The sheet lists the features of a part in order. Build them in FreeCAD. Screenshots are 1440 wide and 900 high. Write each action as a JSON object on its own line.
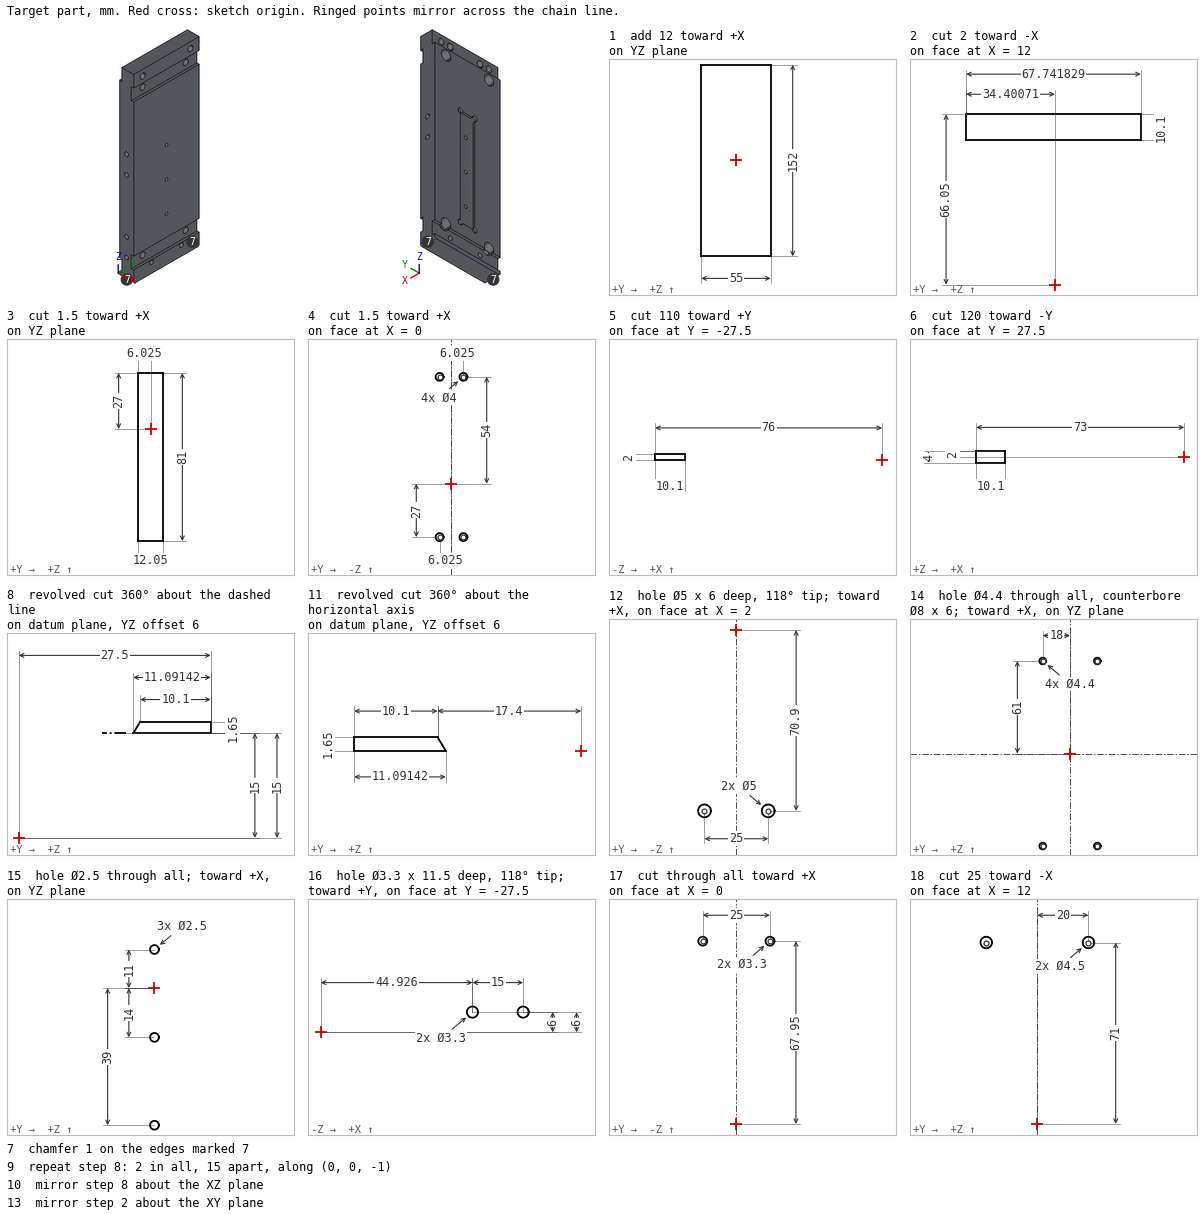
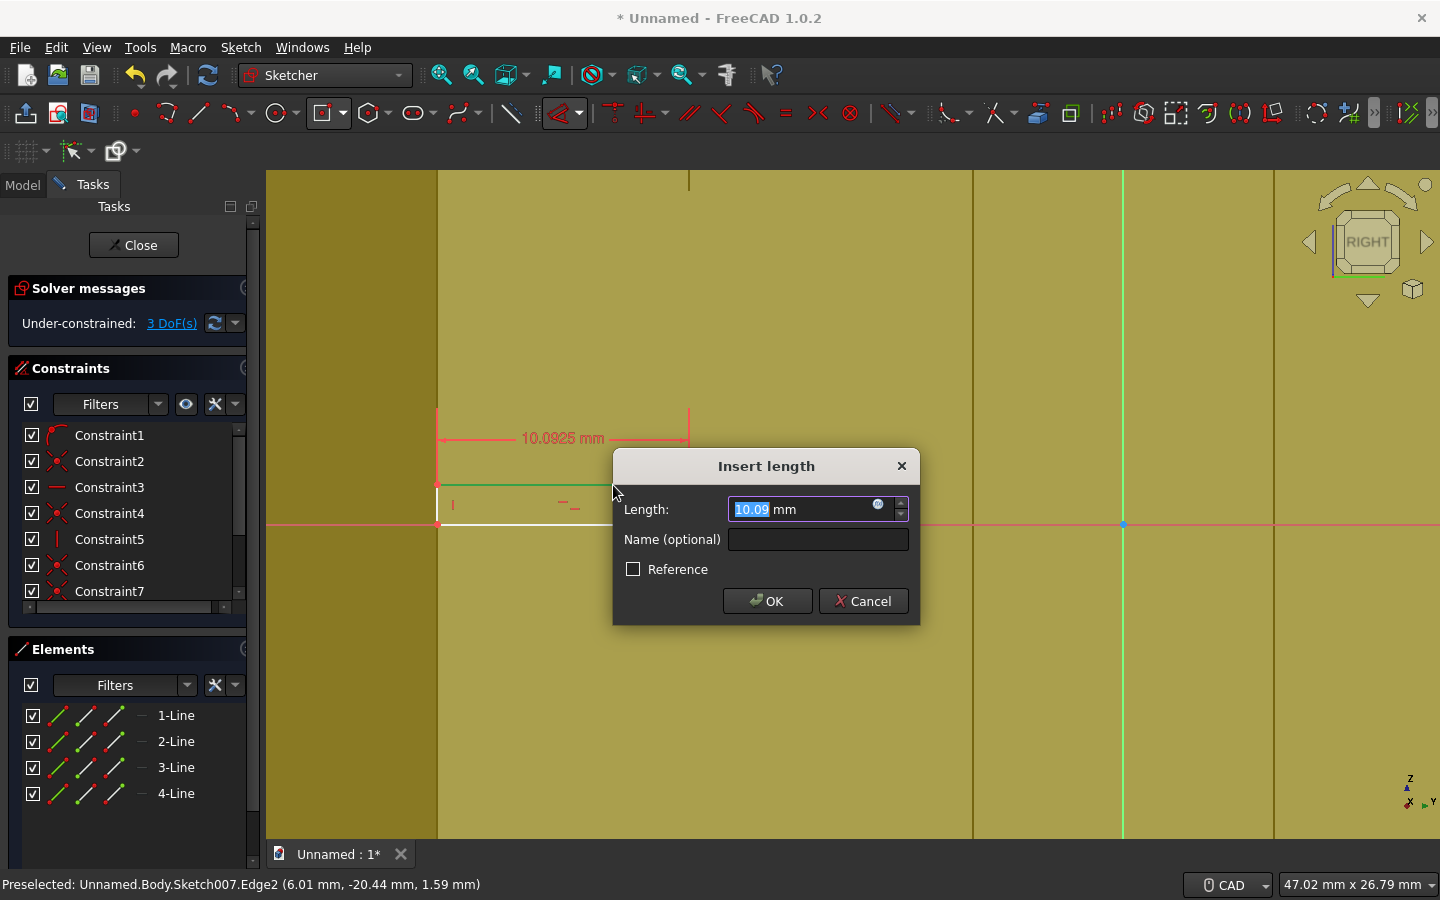
{"action": "type", "text": "10.1"}
{"action": "key", "text": "Return"}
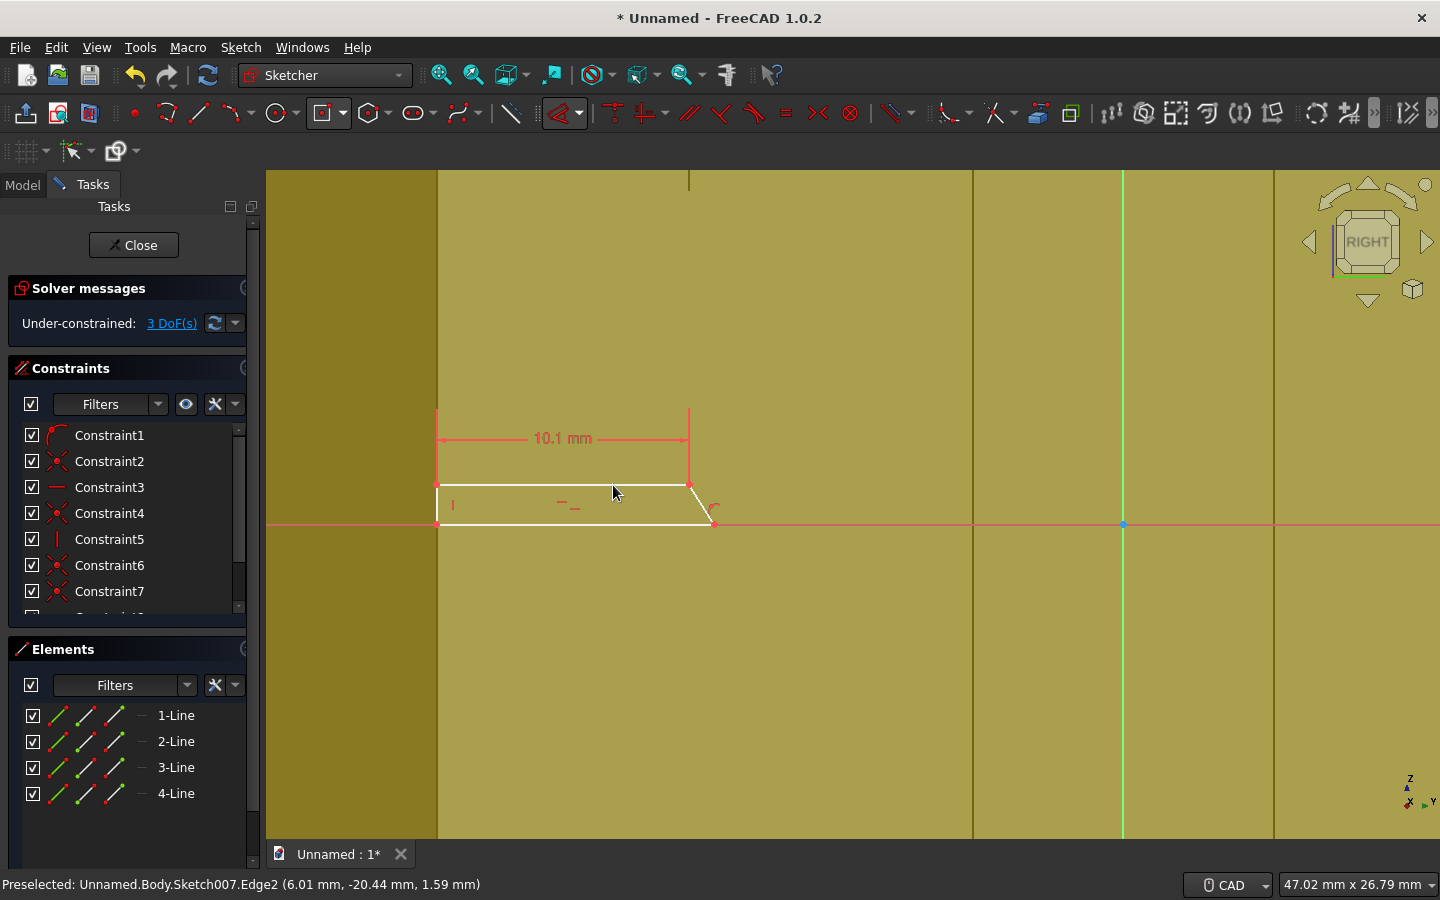
{"action": "left_click", "coordinate": [437, 497]}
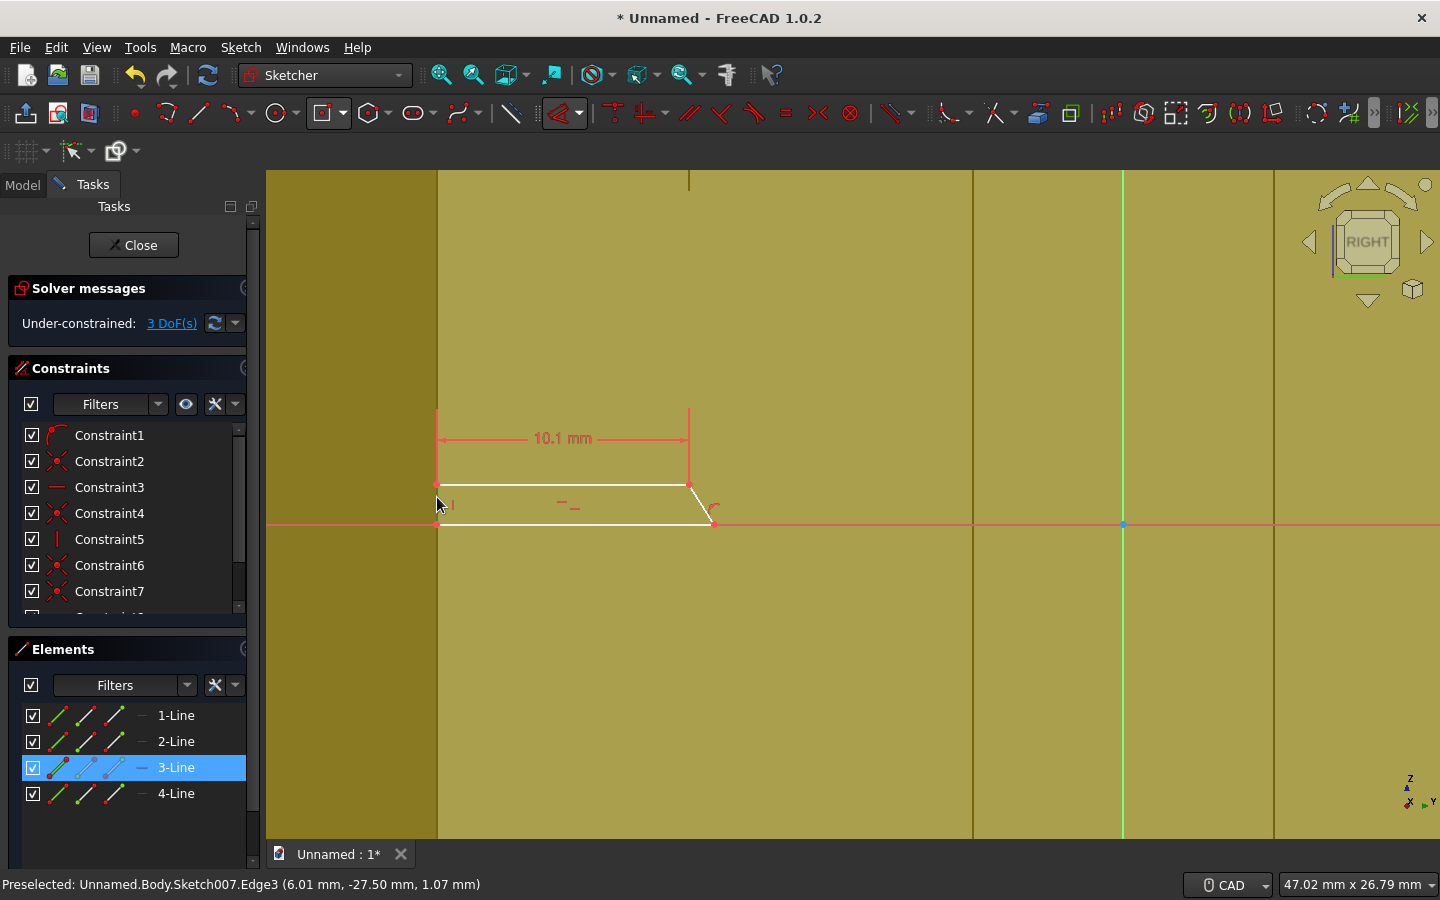
{"action": "key", "text": "i"}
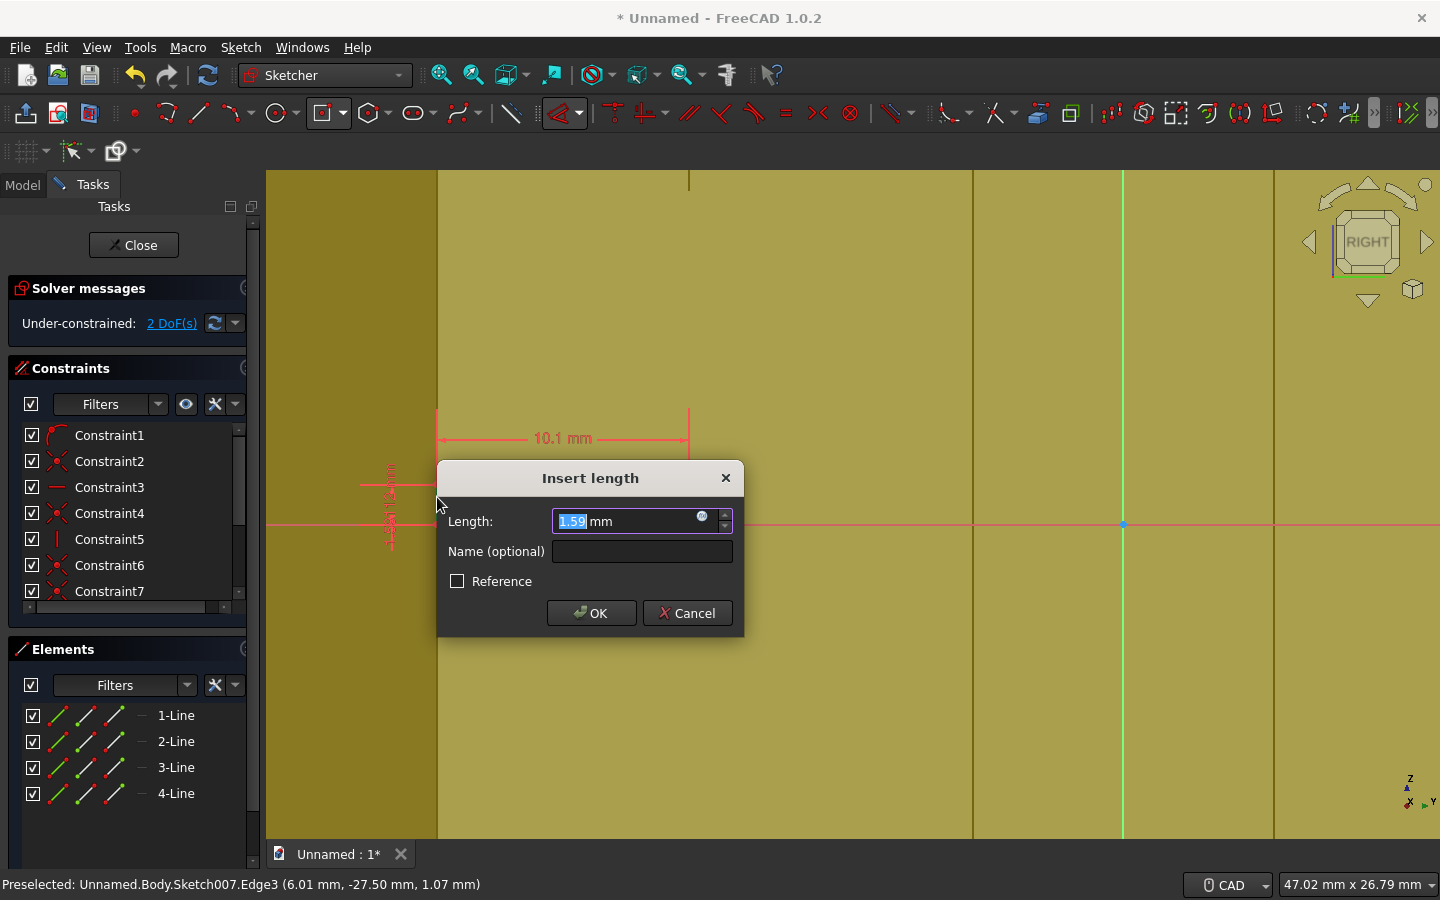
{"action": "type", "text": "1.65"}
{"action": "key", "text": "Return"}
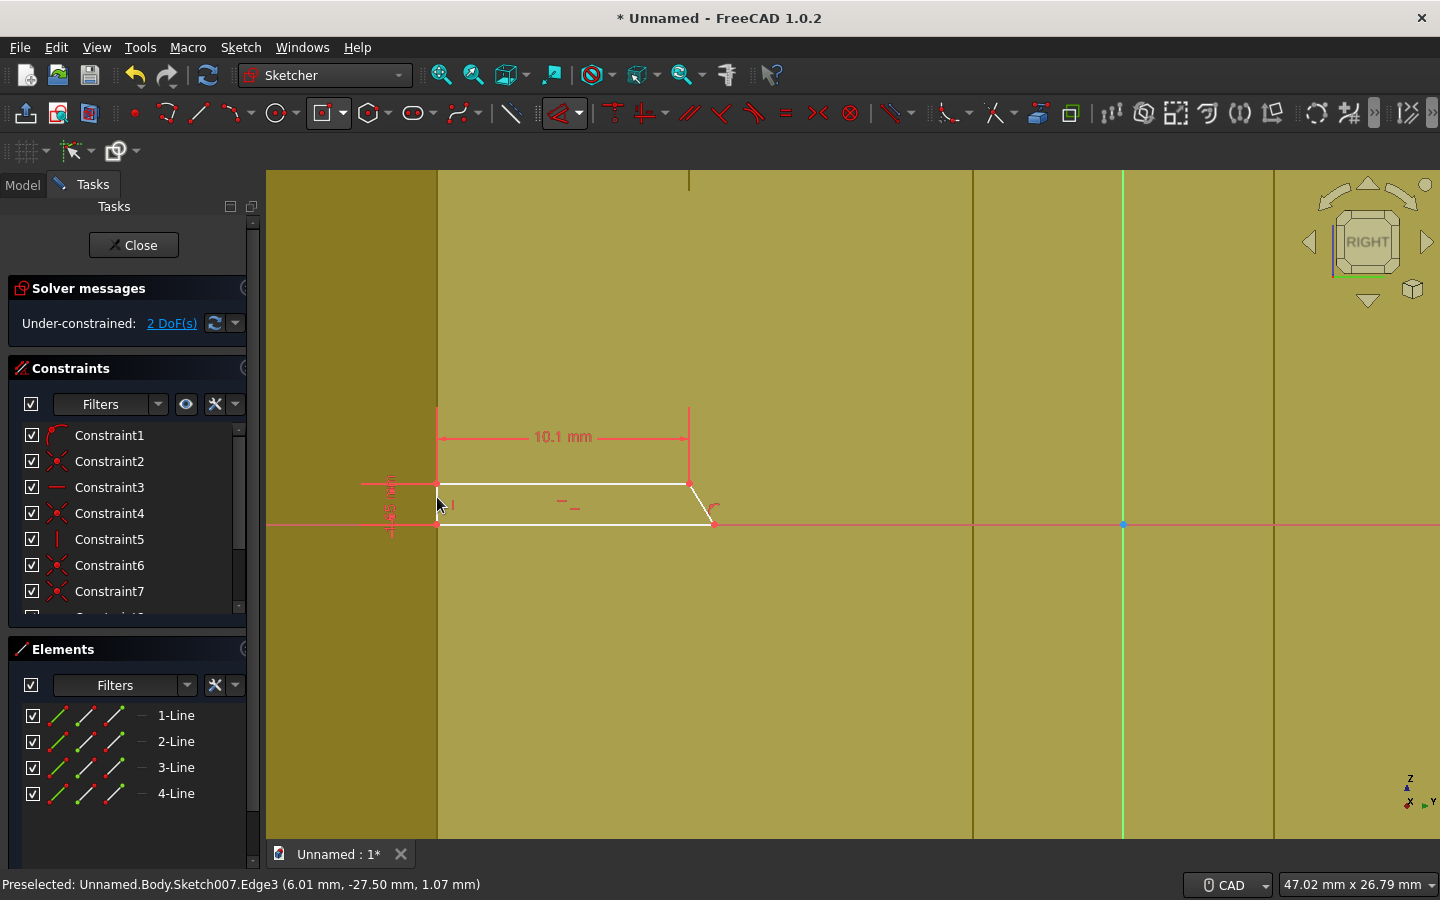
{"action": "left_click", "coordinate": [689, 484]}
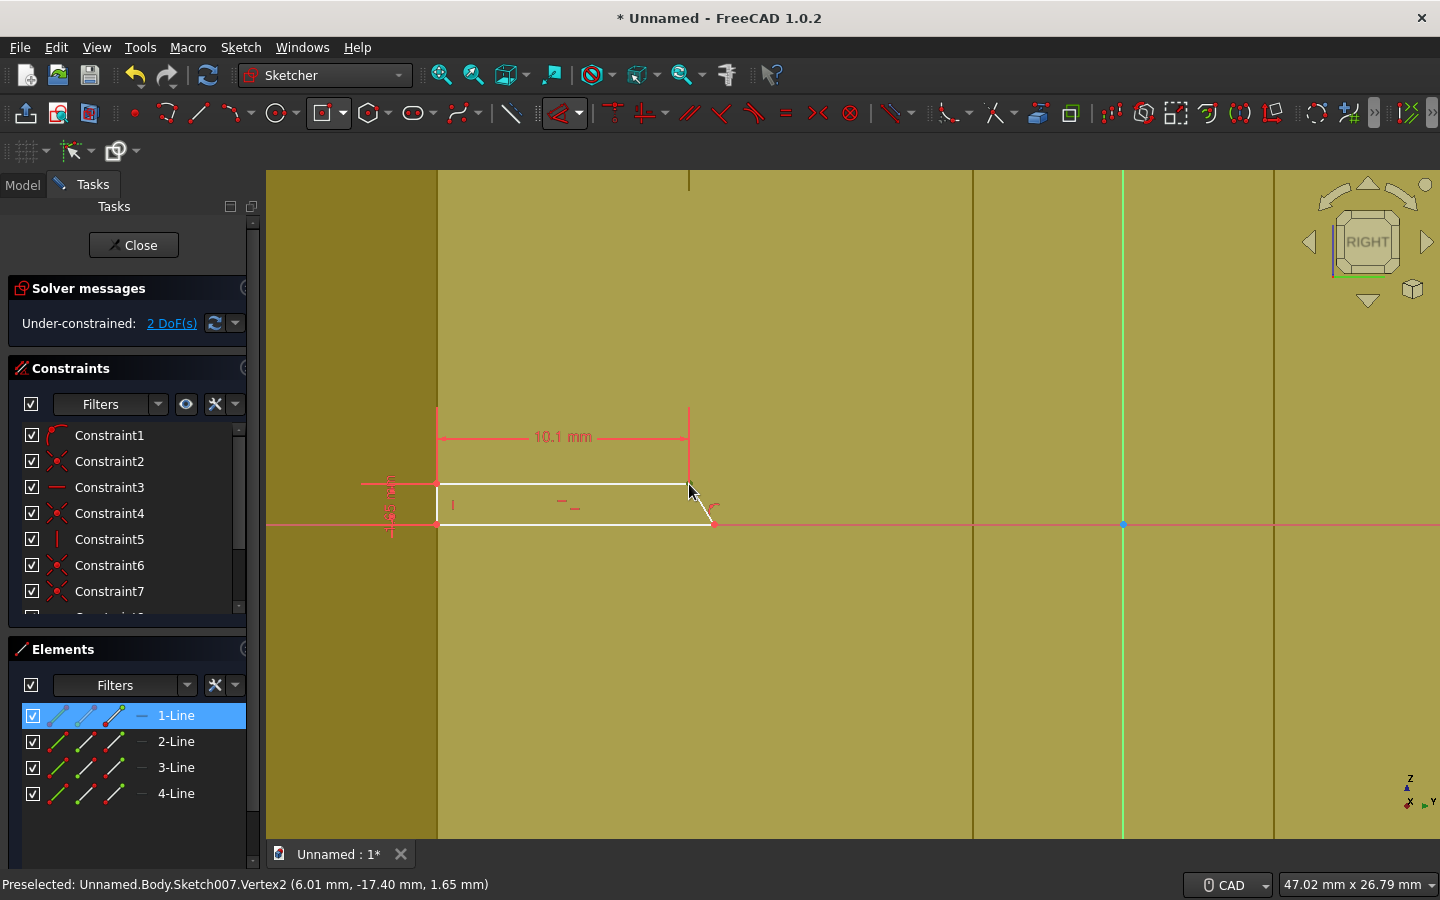
{"action": "left_click", "coordinate": [582, 114]}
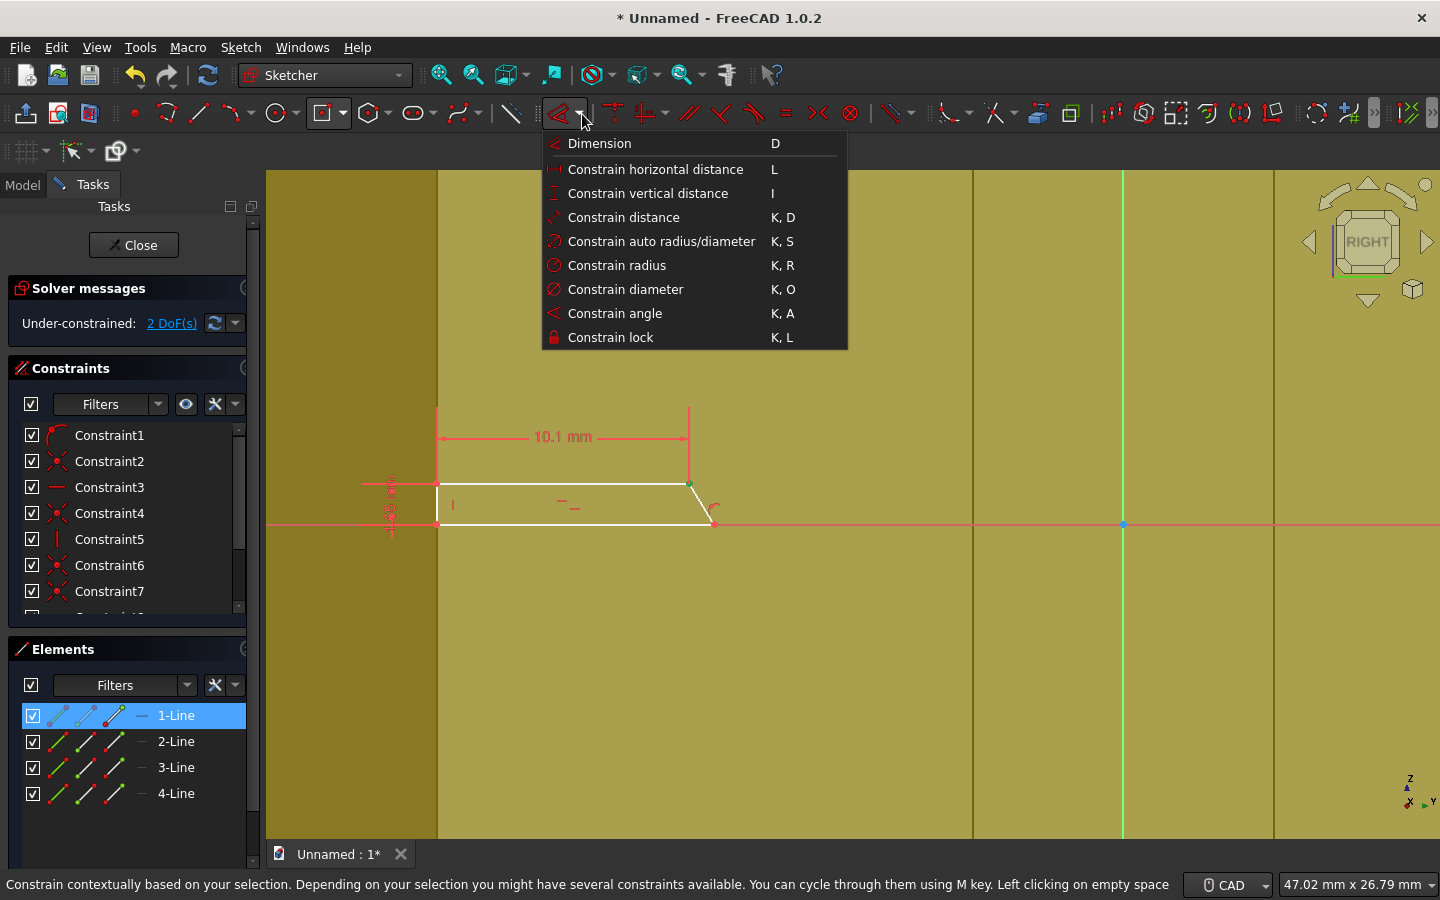
{"action": "left_click", "coordinate": [695, 169]}